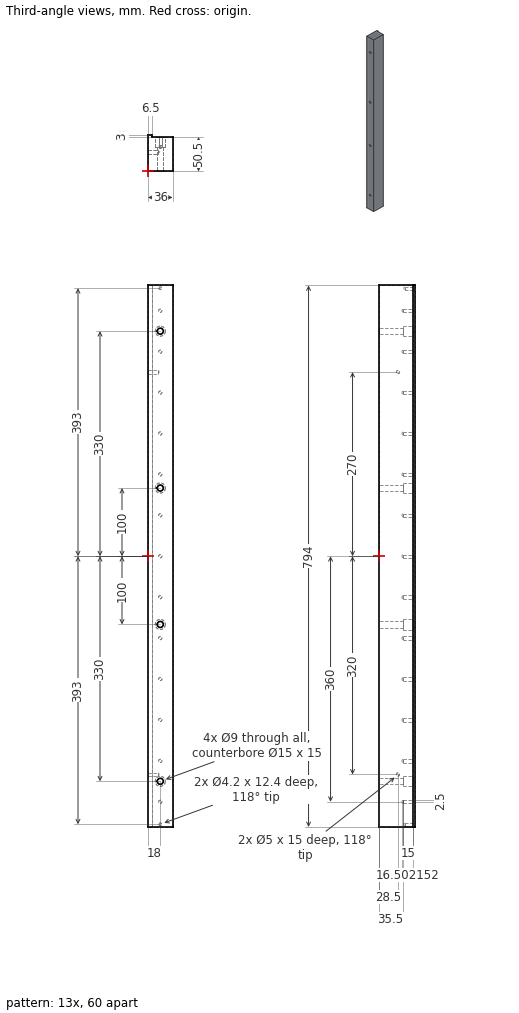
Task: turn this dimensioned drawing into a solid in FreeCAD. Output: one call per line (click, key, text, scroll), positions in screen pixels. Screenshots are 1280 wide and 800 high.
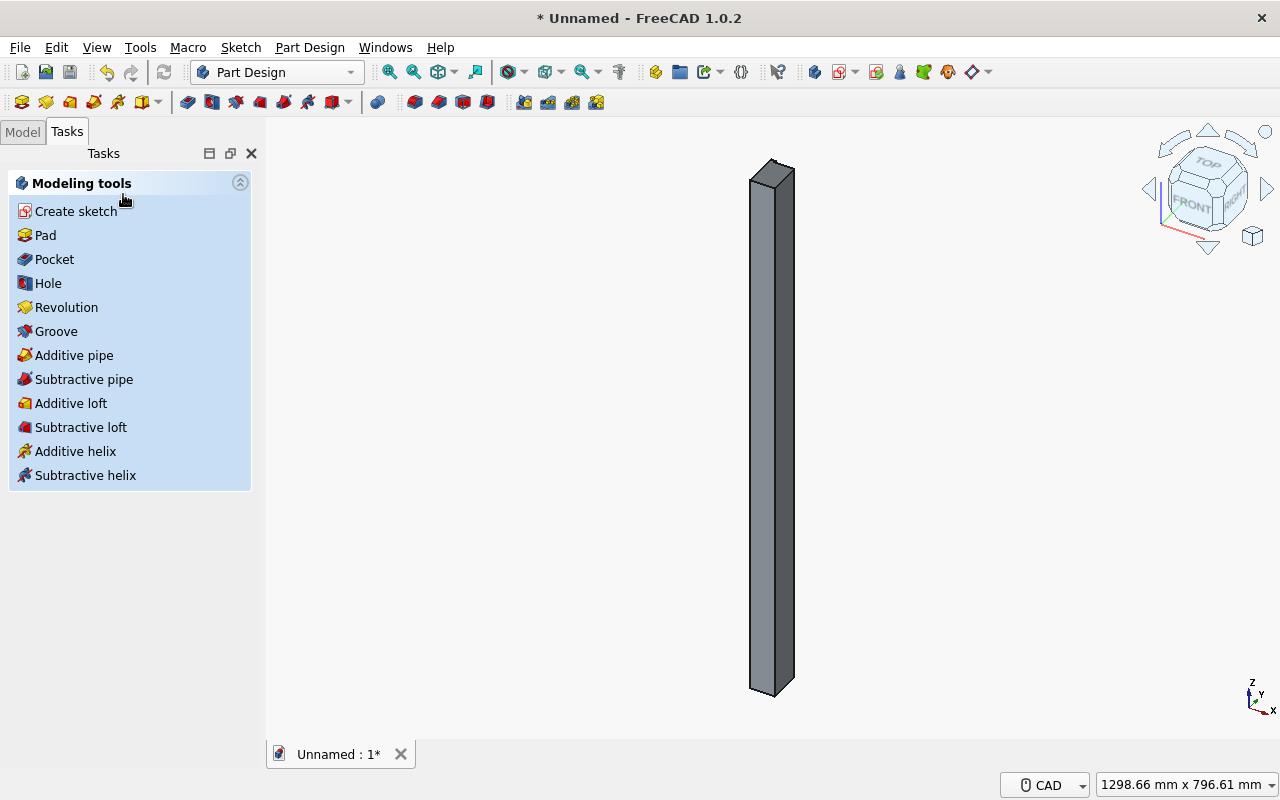
click(212, 102)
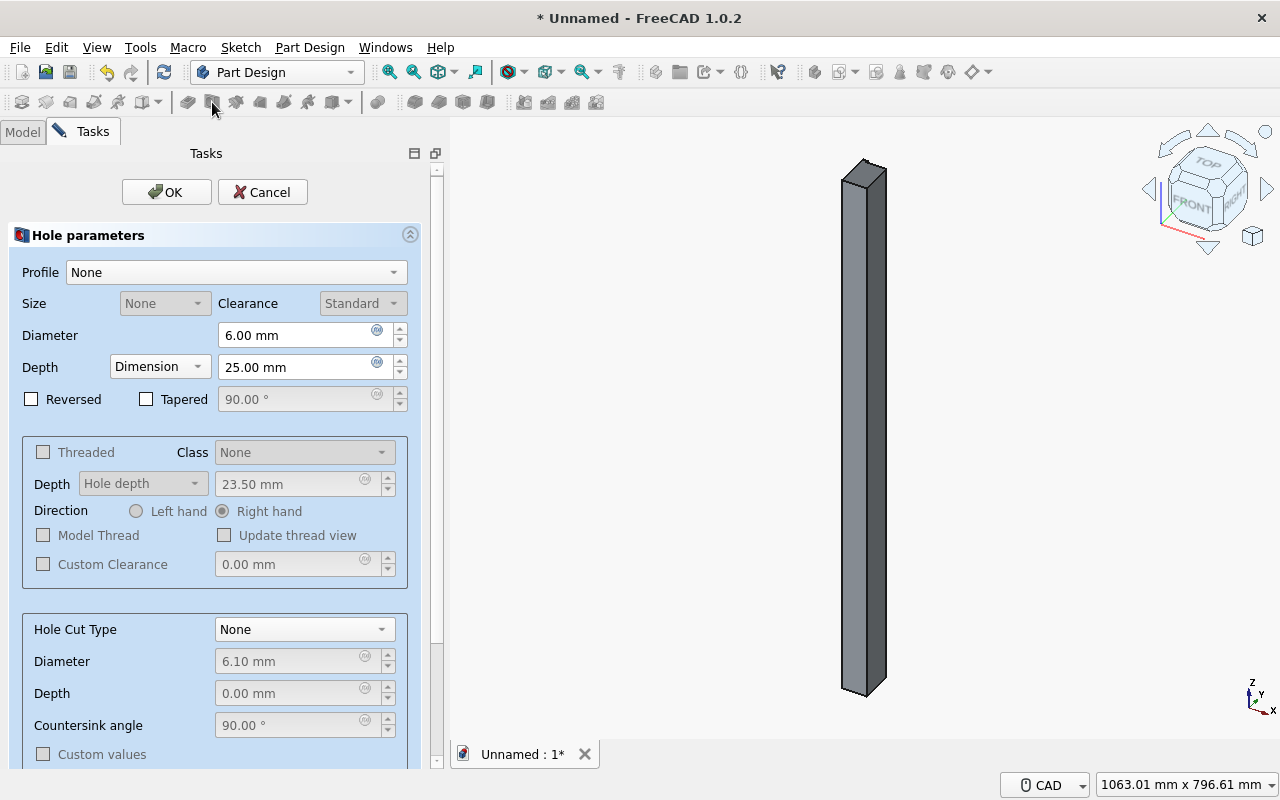
triple_click(305, 335)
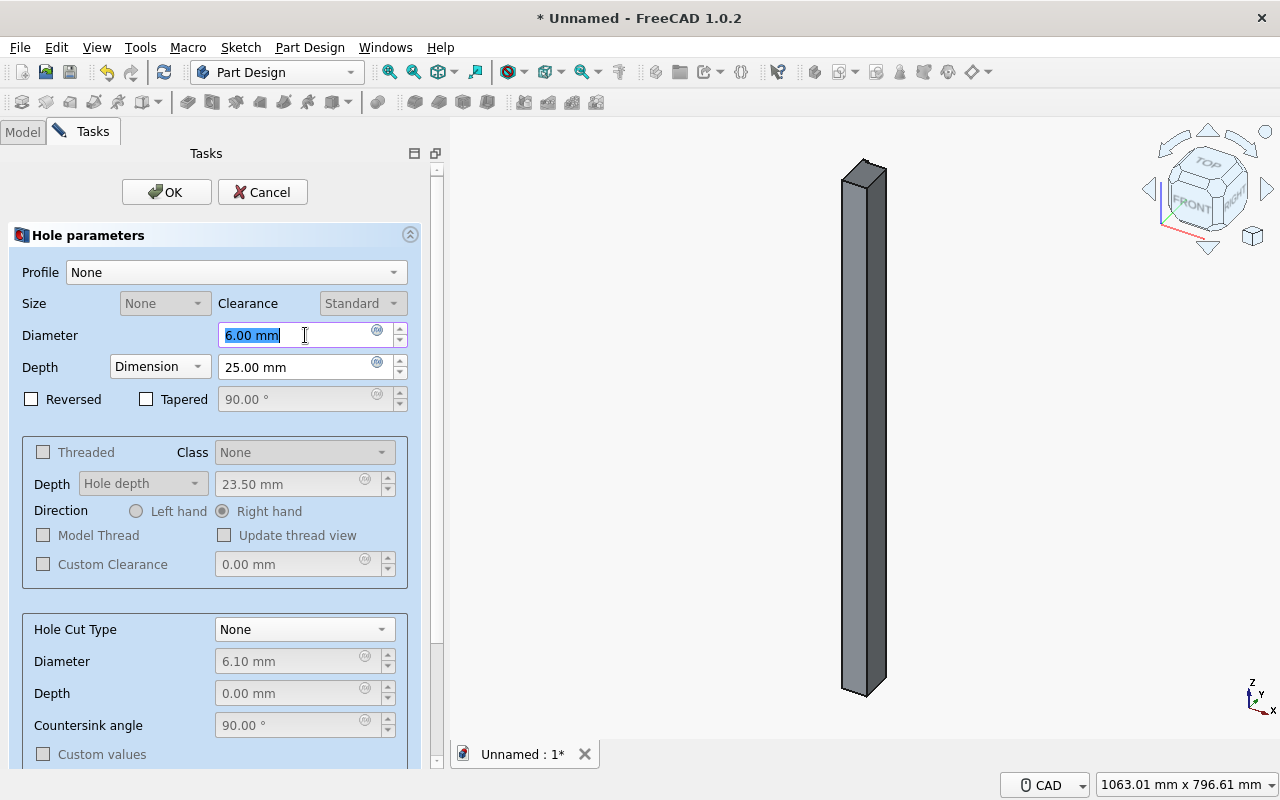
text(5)
key(Tab)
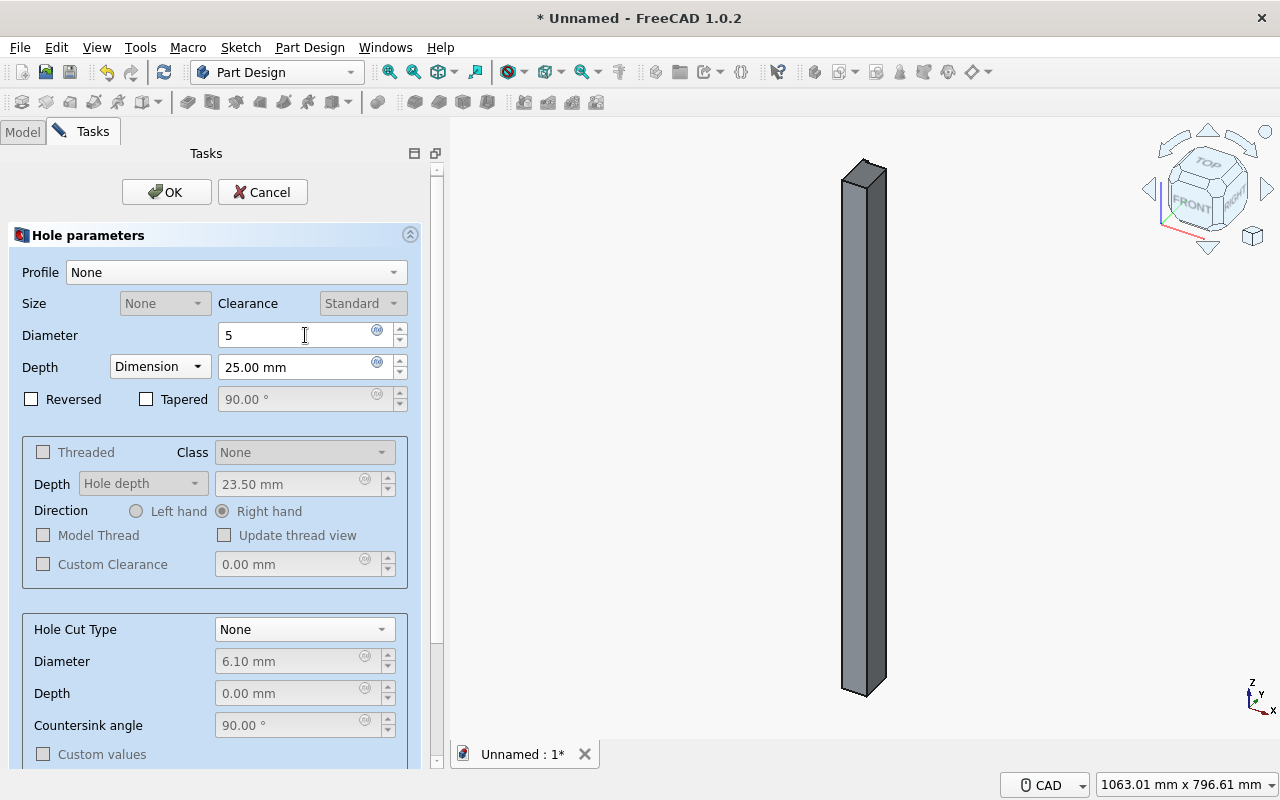
triple_click(305, 367)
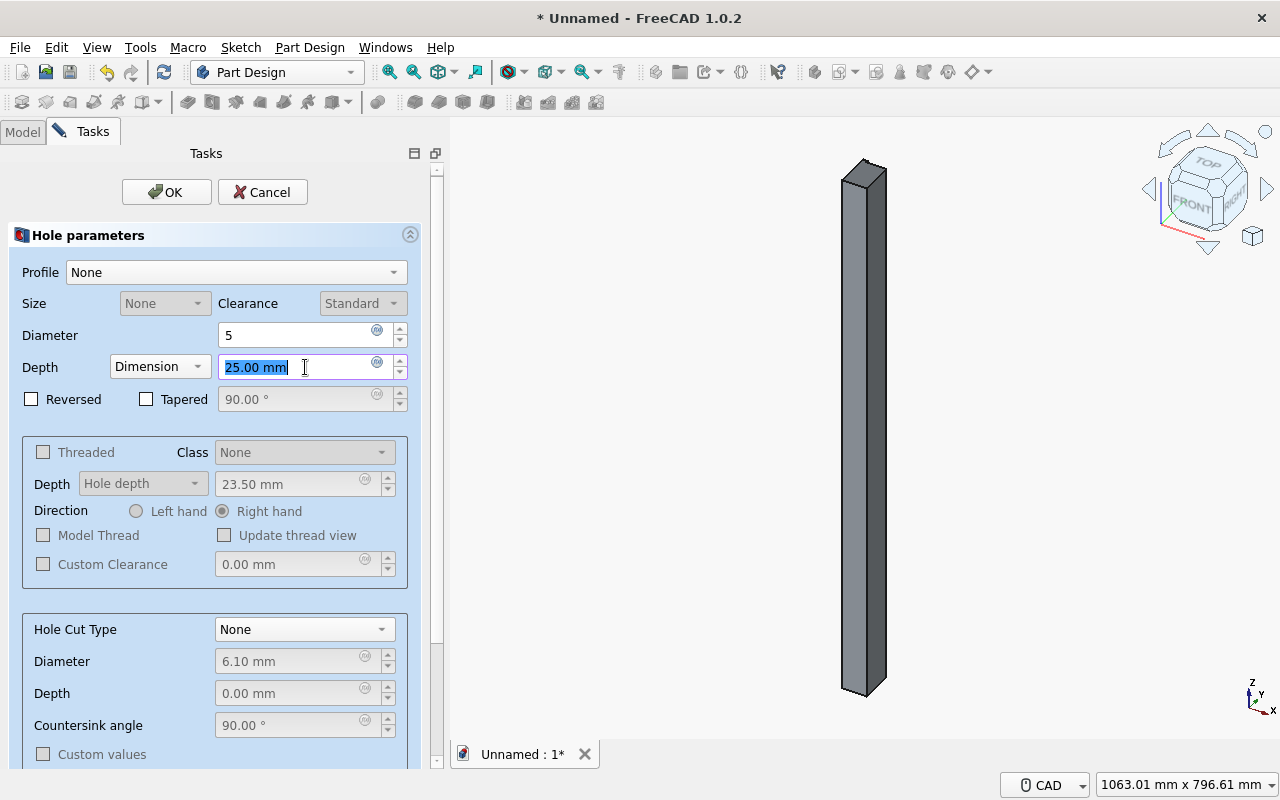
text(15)
key(Tab)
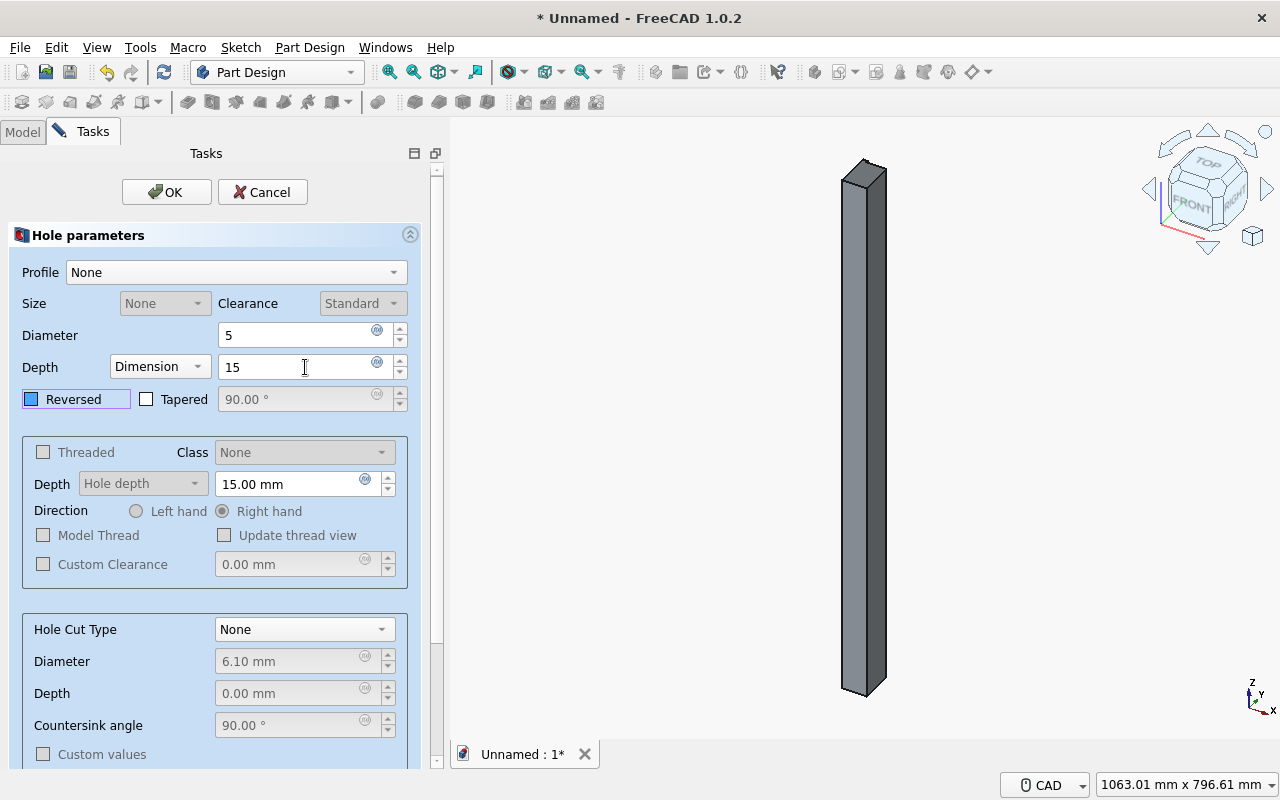
click(30, 399)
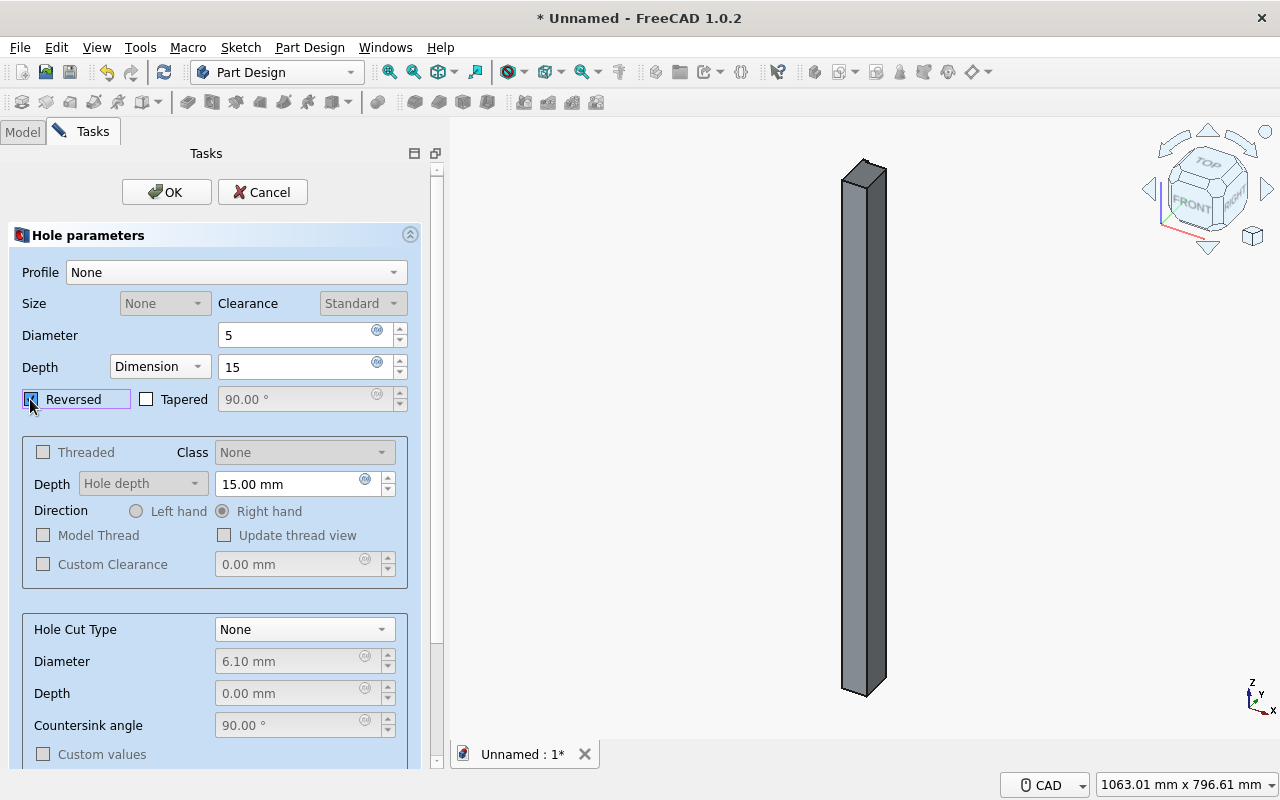
click(167, 192)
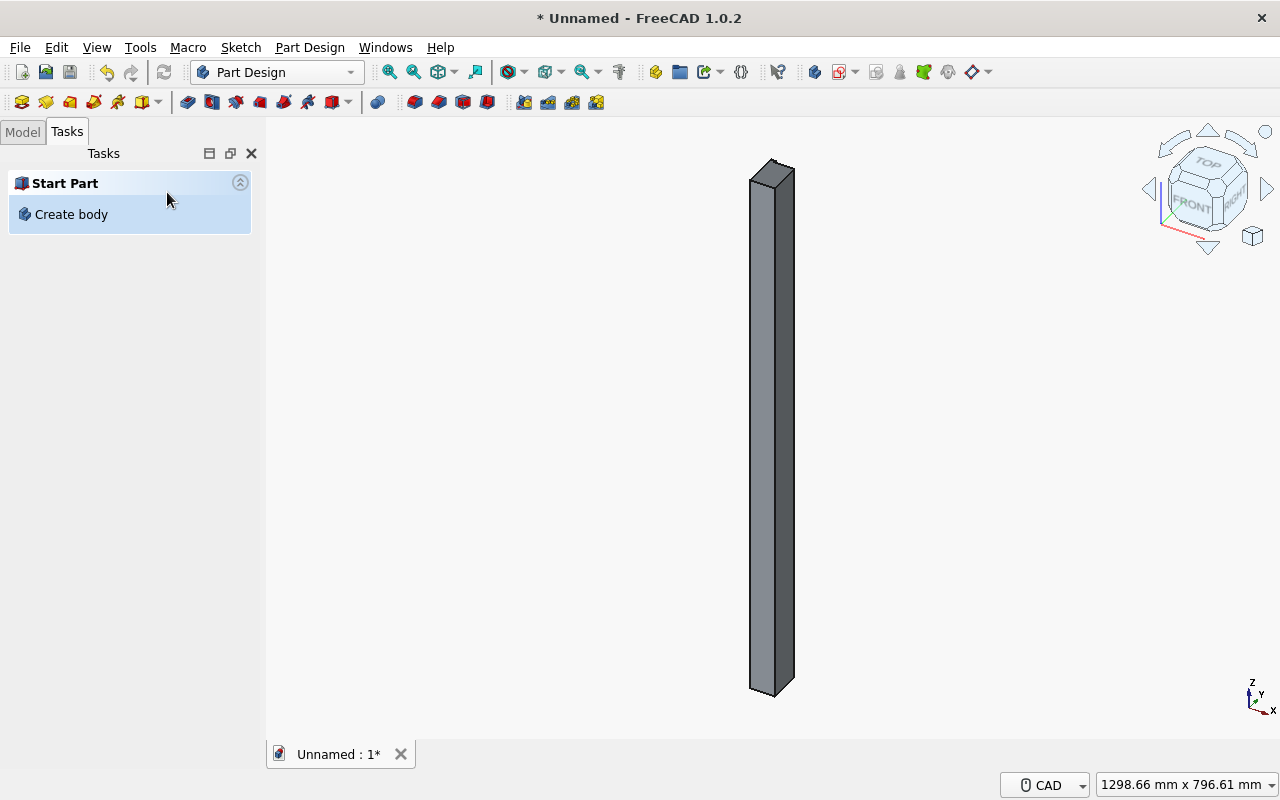
click(23, 131)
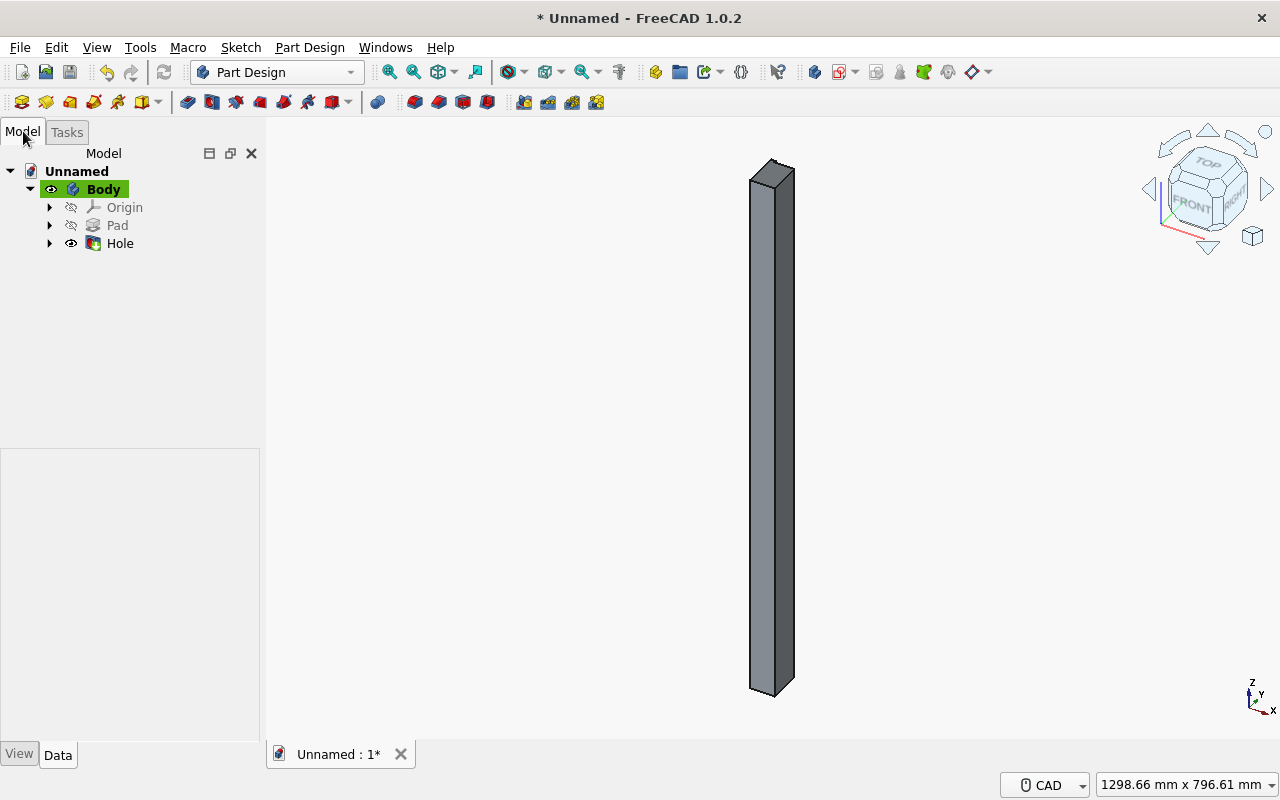
click(50, 207)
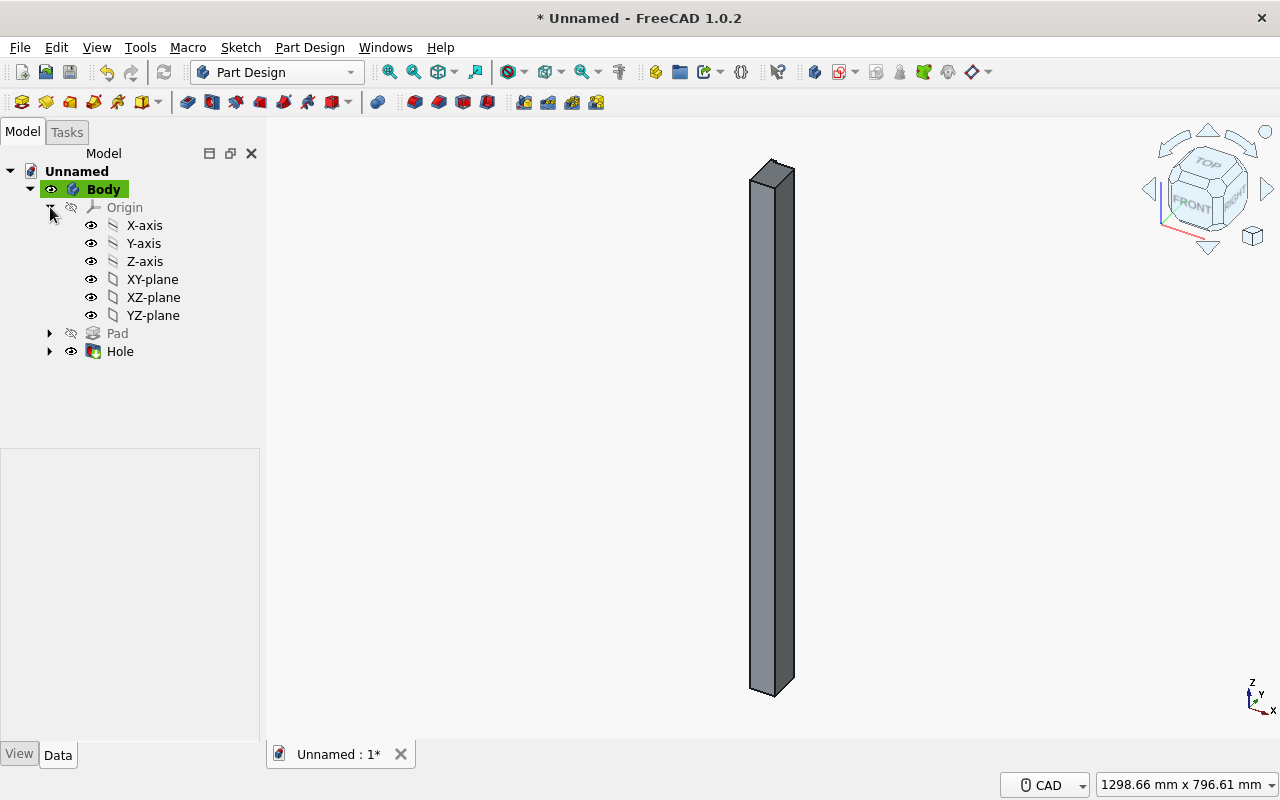
click(136, 315)